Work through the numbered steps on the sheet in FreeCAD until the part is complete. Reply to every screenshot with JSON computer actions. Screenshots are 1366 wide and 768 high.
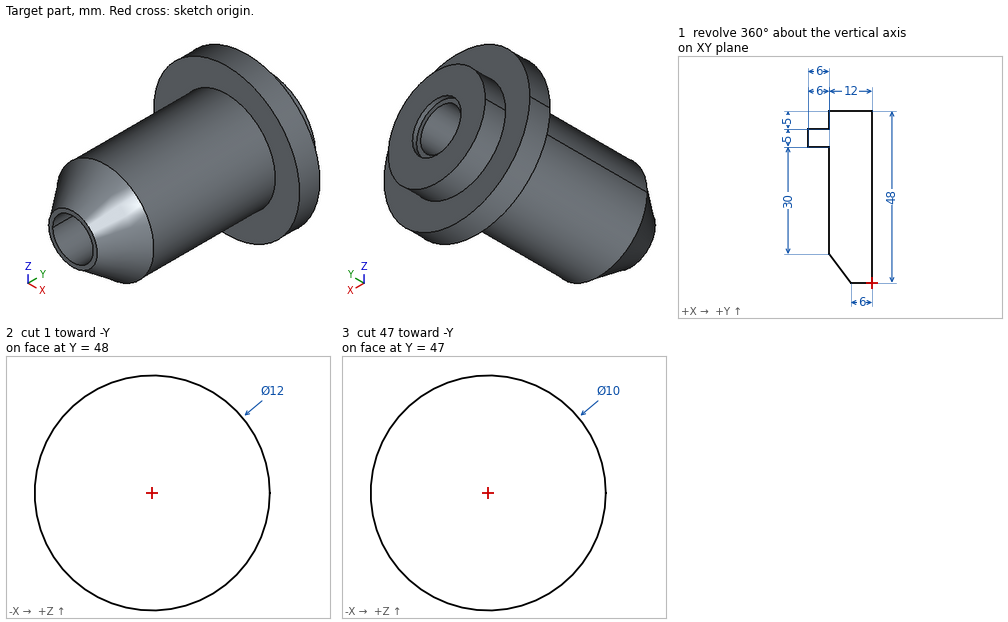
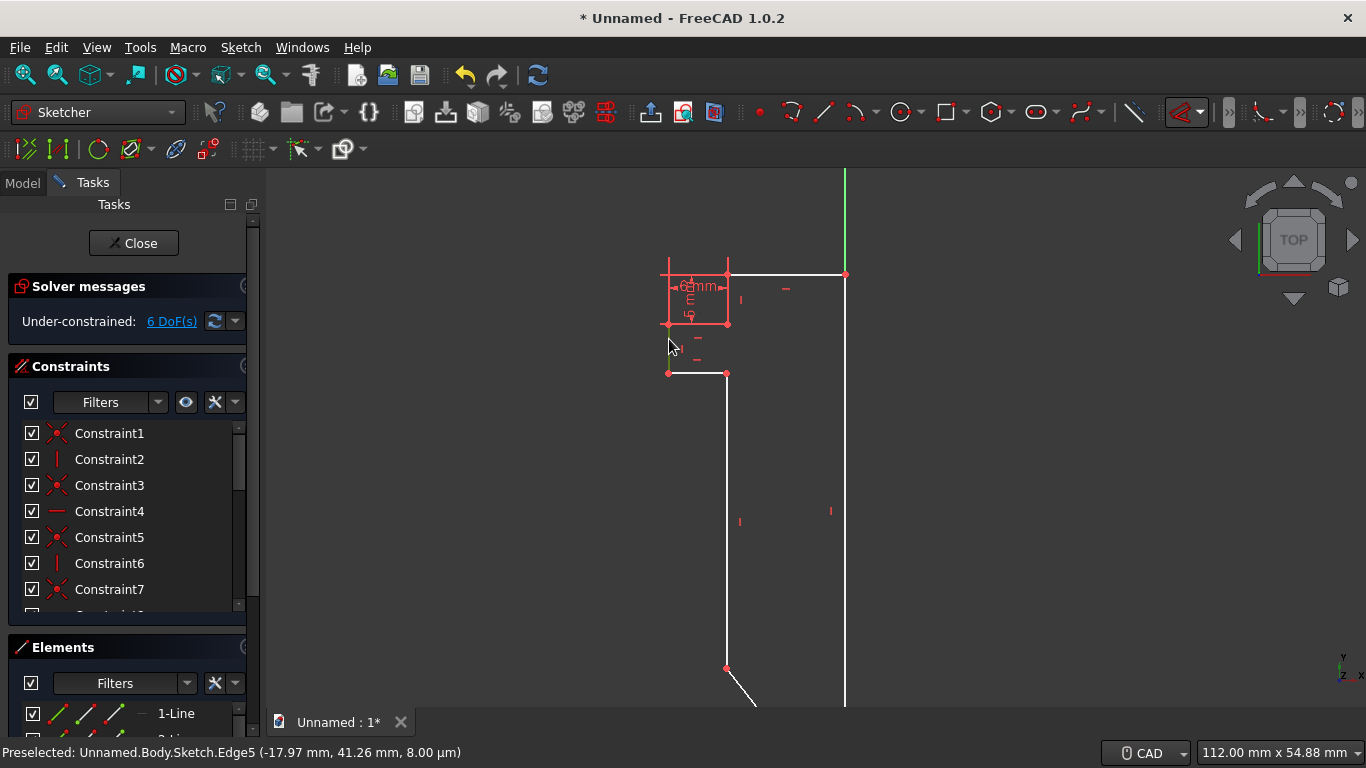
{"action": "left_click", "coordinate": [1202, 112]}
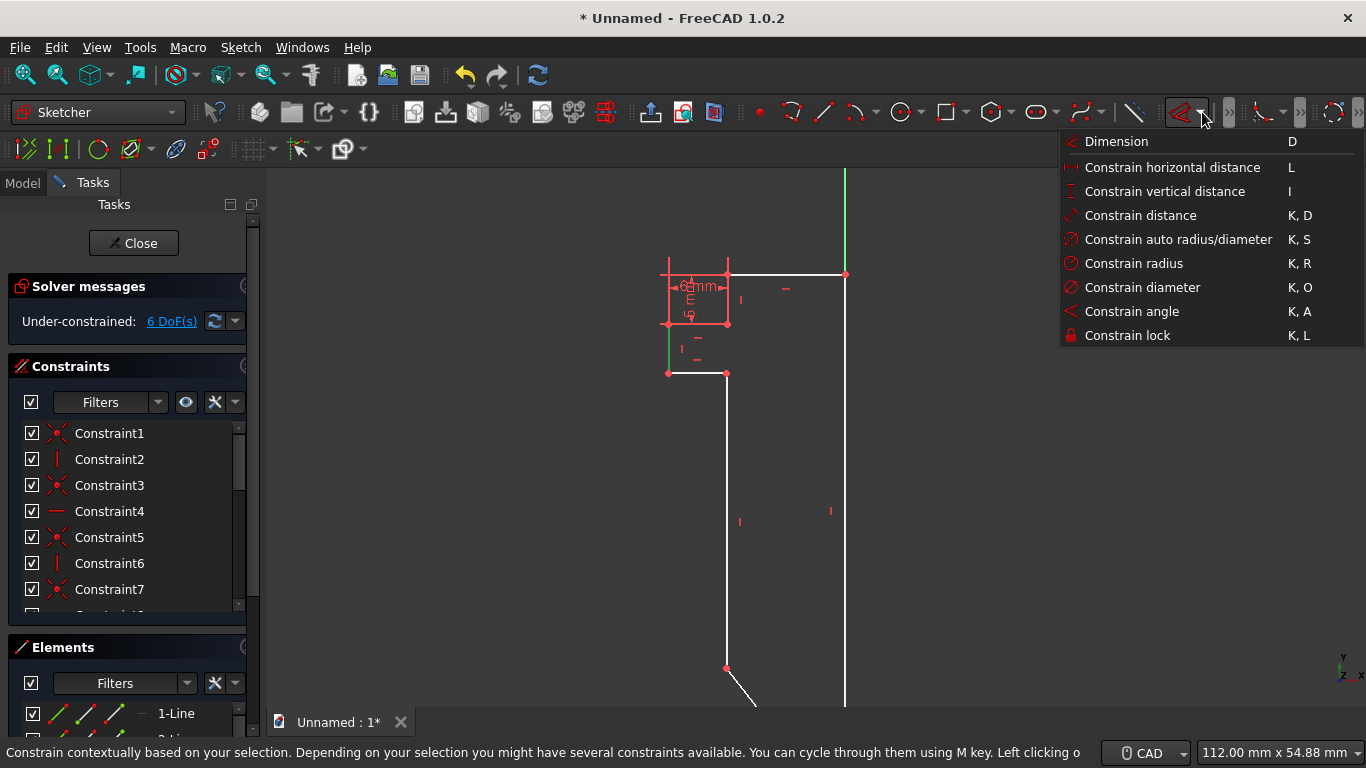
{"action": "left_click", "coordinate": [1212, 191]}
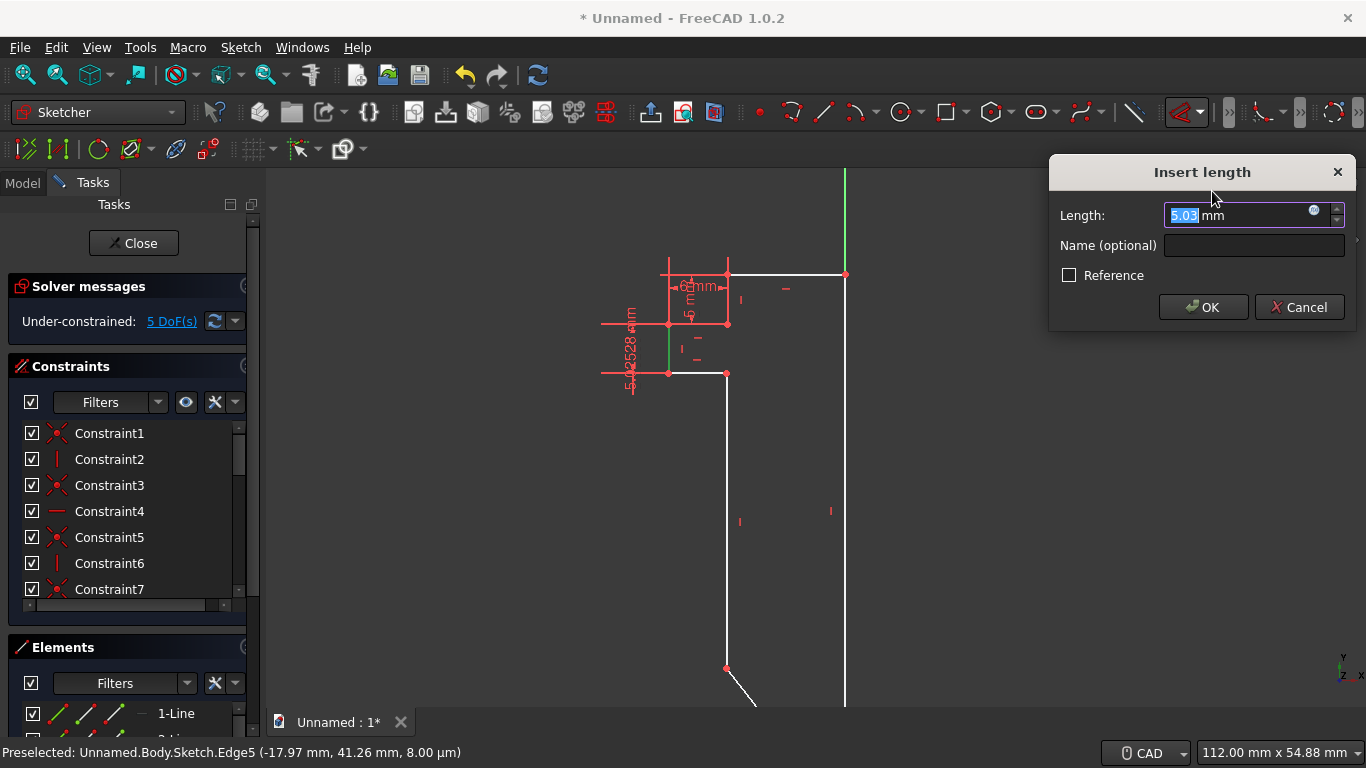
{"action": "type", "text": "5"}
{"action": "key", "text": "Return"}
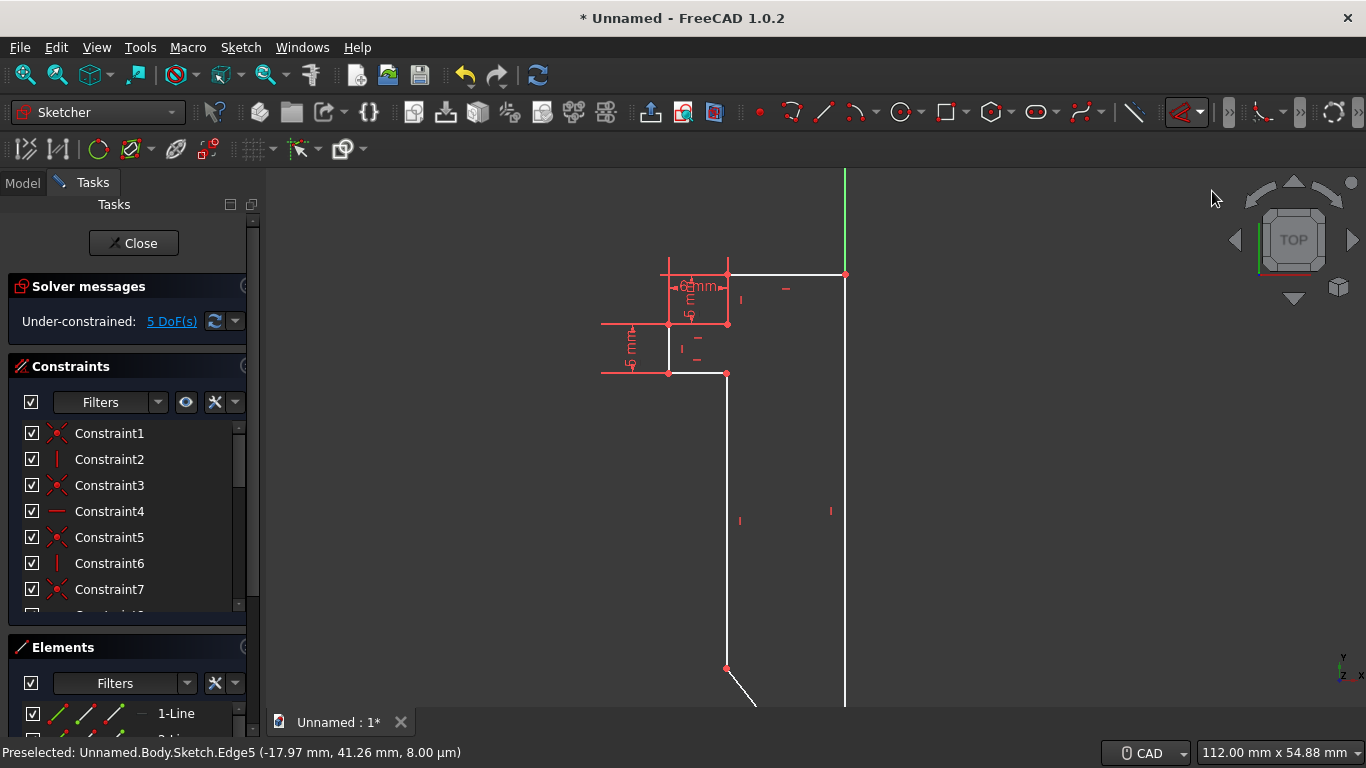
{"action": "left_click", "coordinate": [686, 373]}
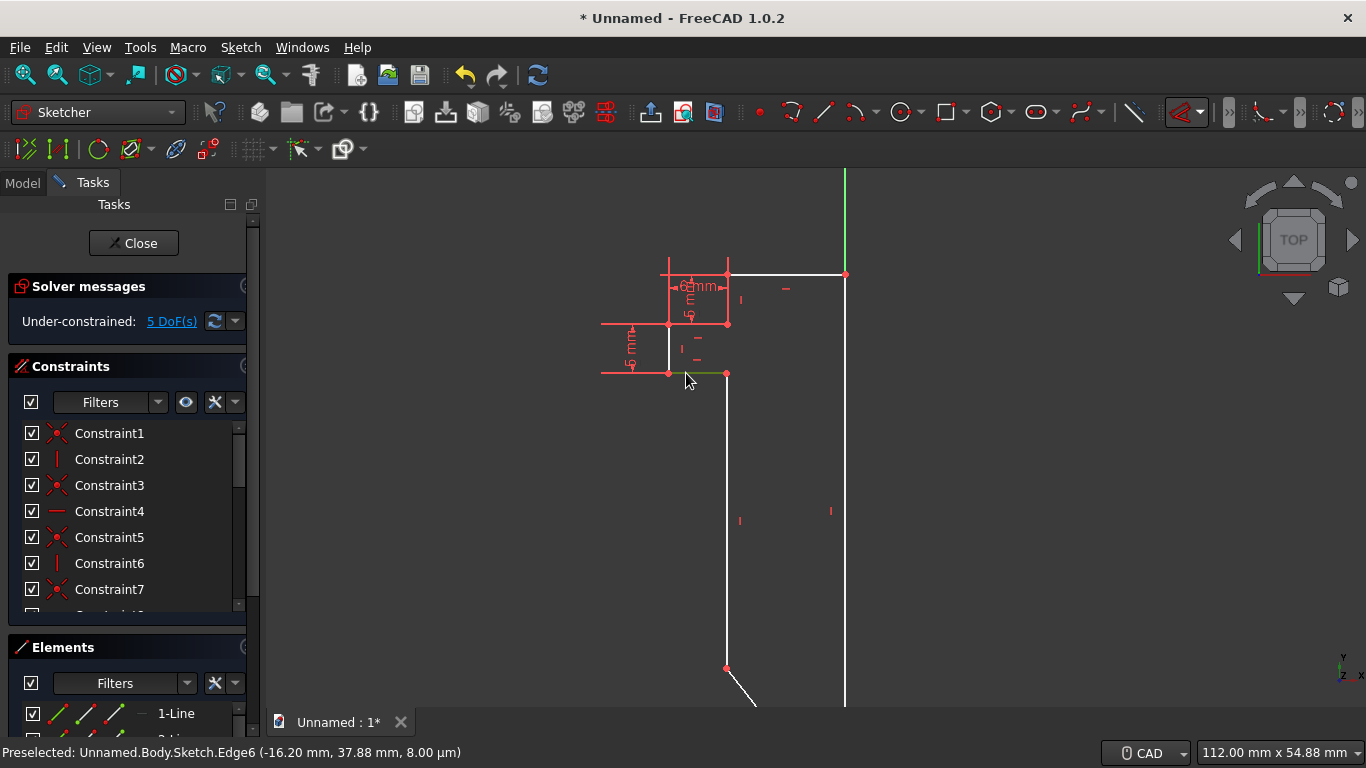
{"action": "key", "text": "l"}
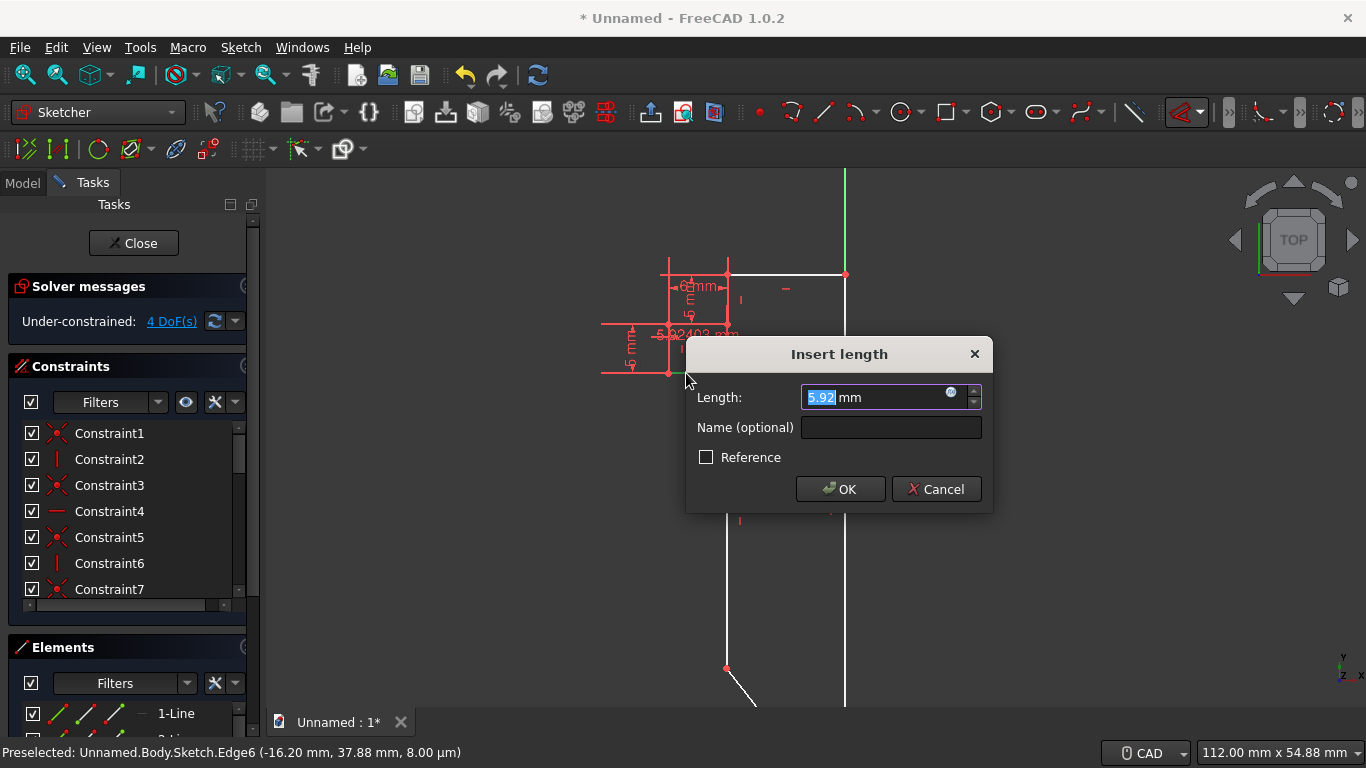
{"action": "type", "text": "6"}
{"action": "key", "text": "Return"}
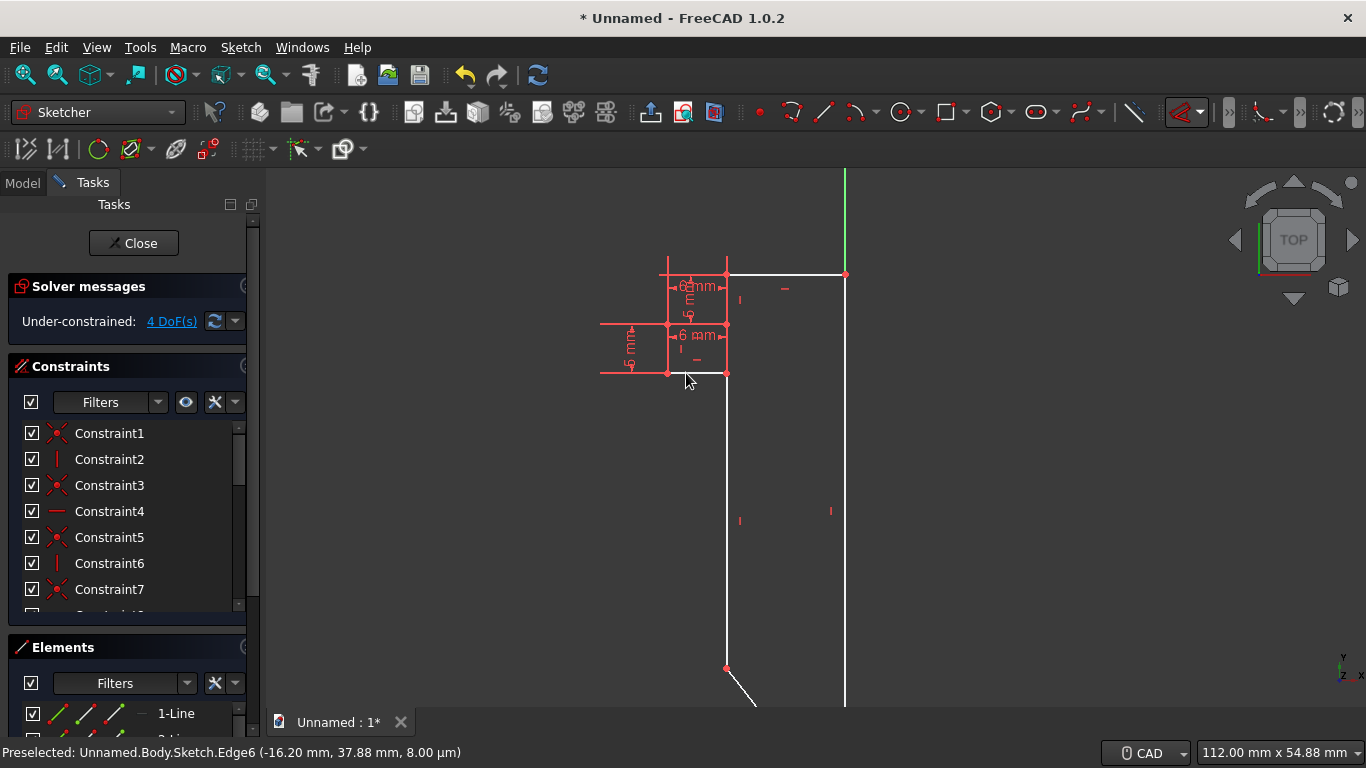
{"action": "scroll", "coordinate": [729, 291], "scroll_direction": "down", "scroll_amount": 2}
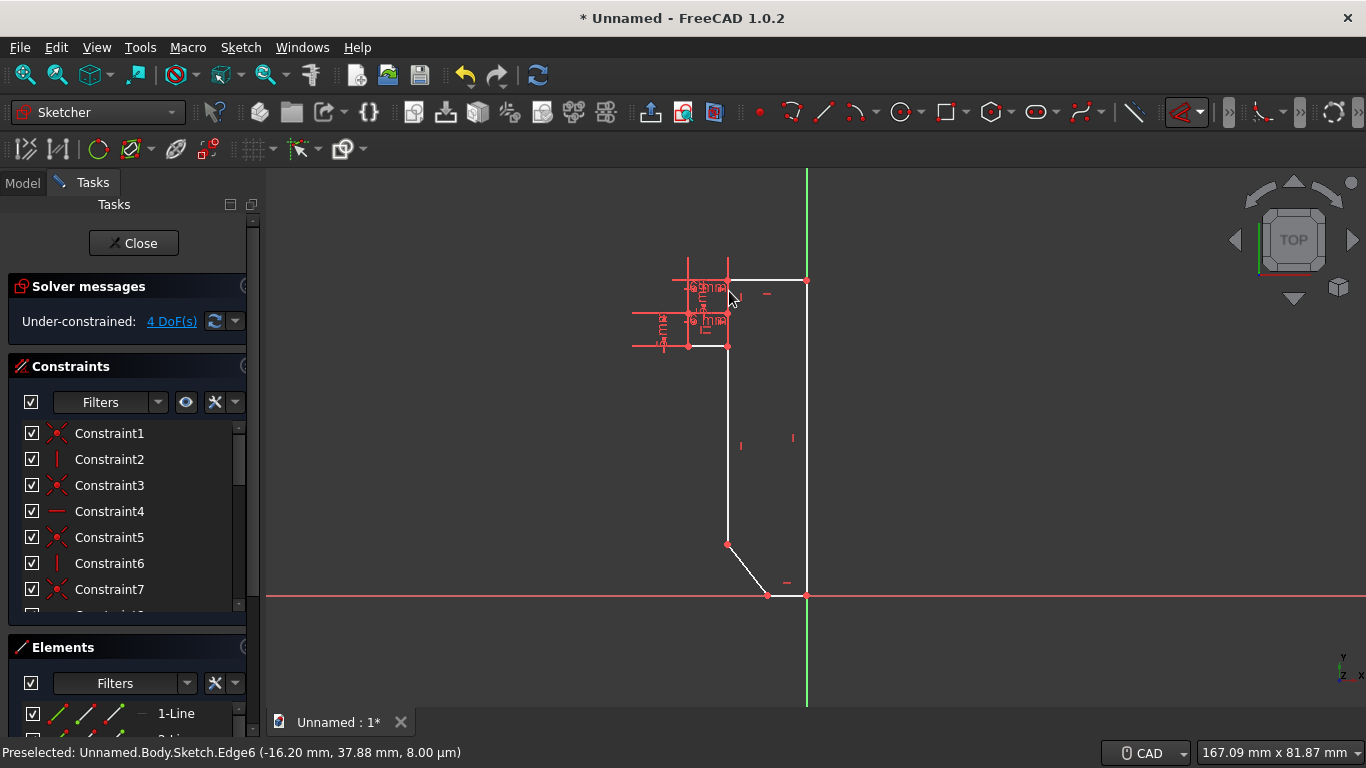
{"action": "left_click", "coordinate": [779, 596]}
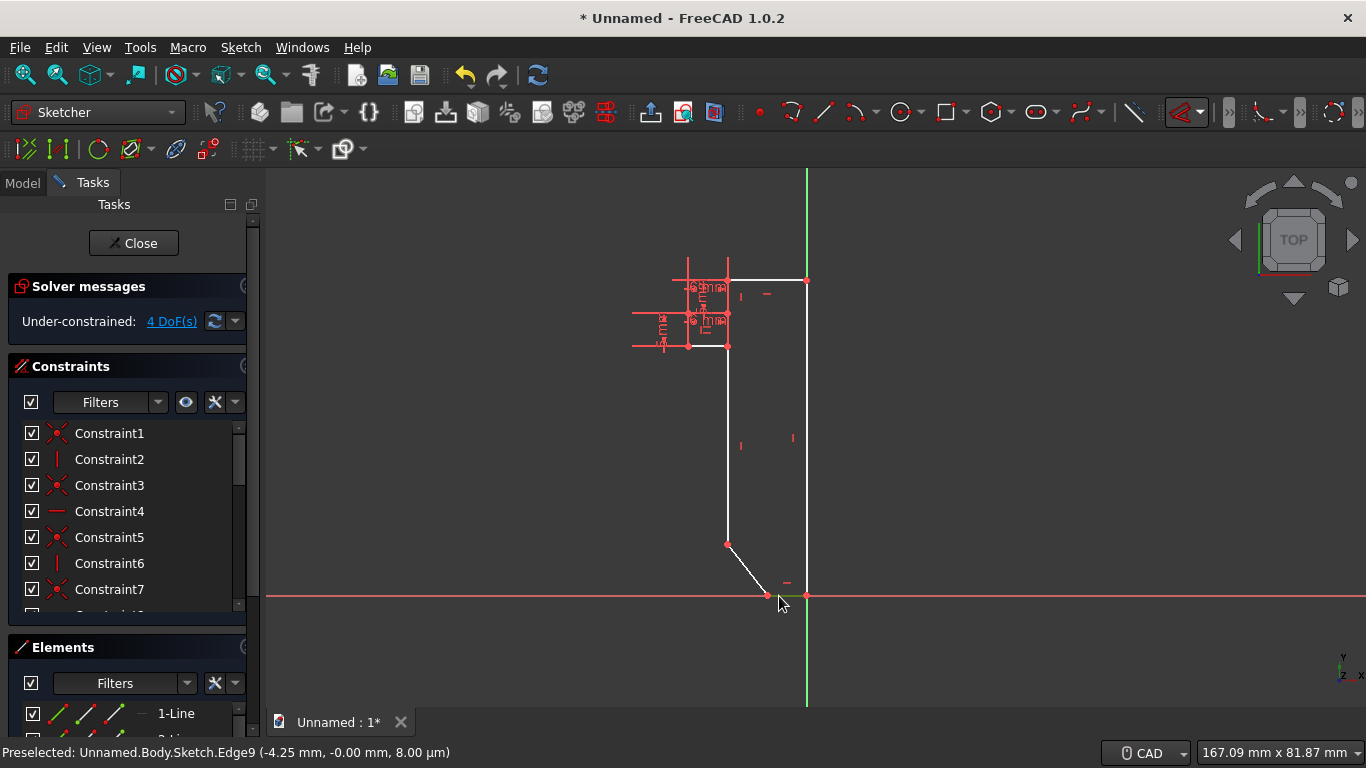
{"action": "key", "text": "l"}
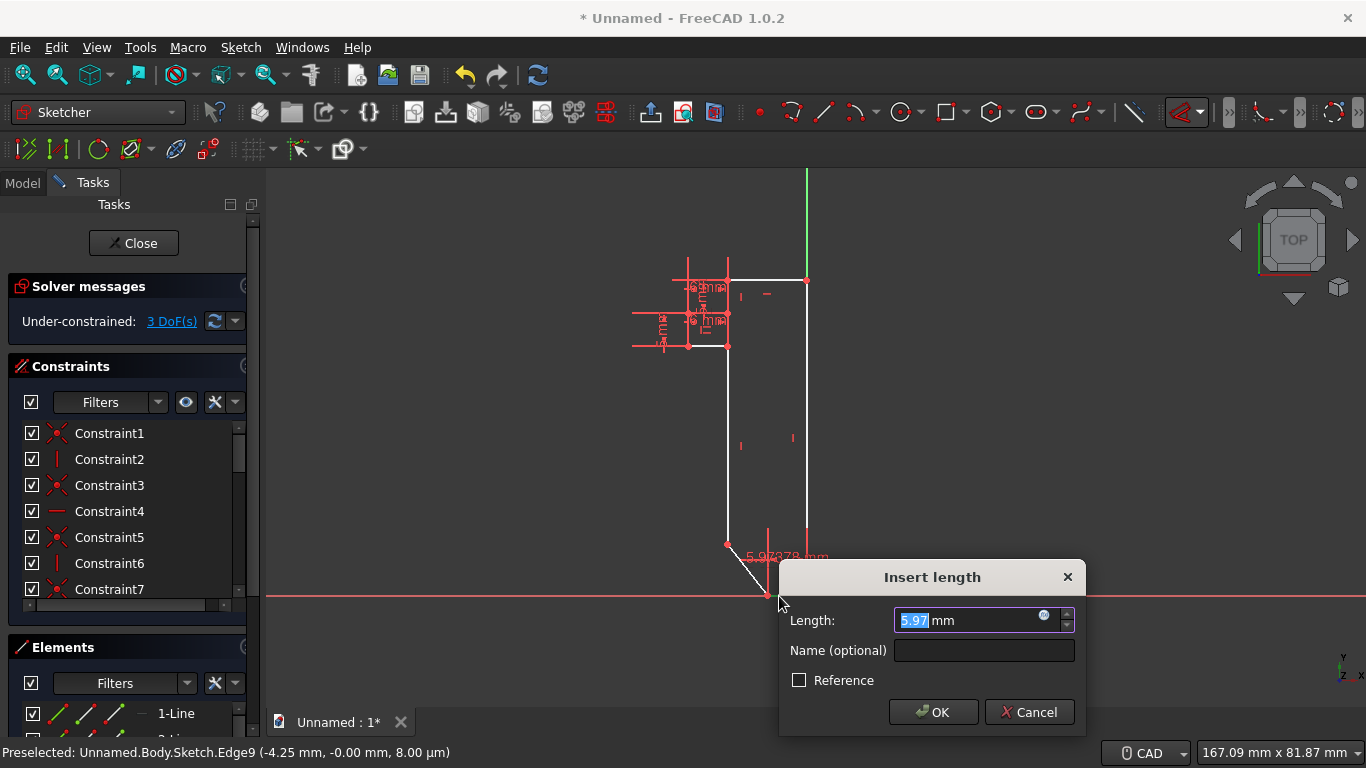
{"action": "type", "text": "6"}
{"action": "key", "text": "Return"}